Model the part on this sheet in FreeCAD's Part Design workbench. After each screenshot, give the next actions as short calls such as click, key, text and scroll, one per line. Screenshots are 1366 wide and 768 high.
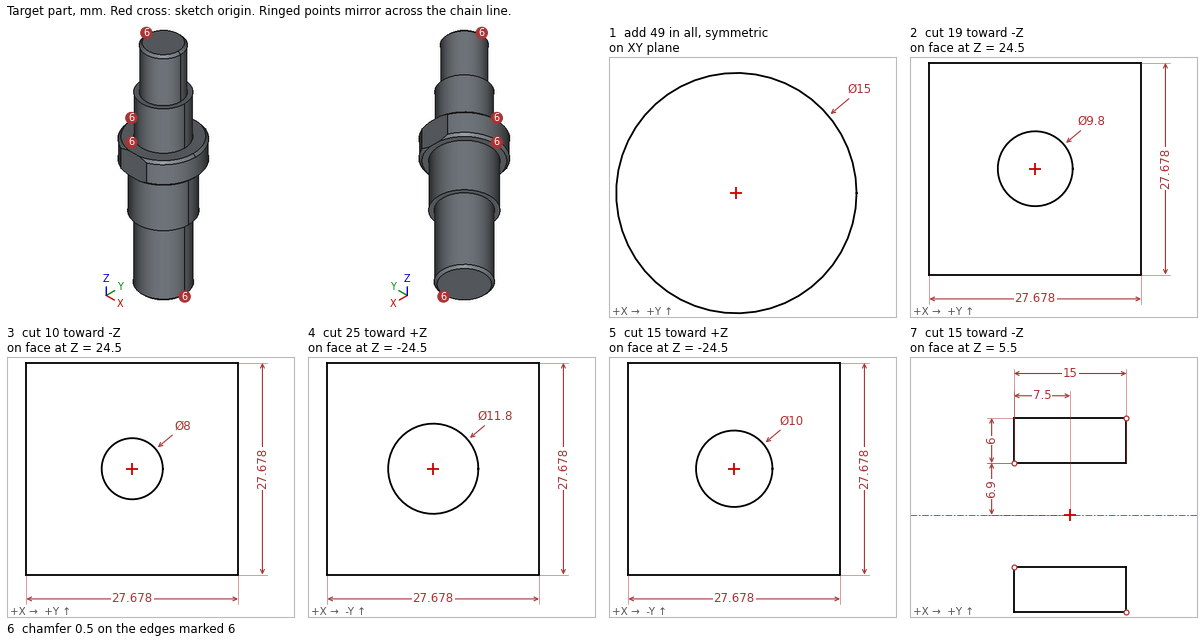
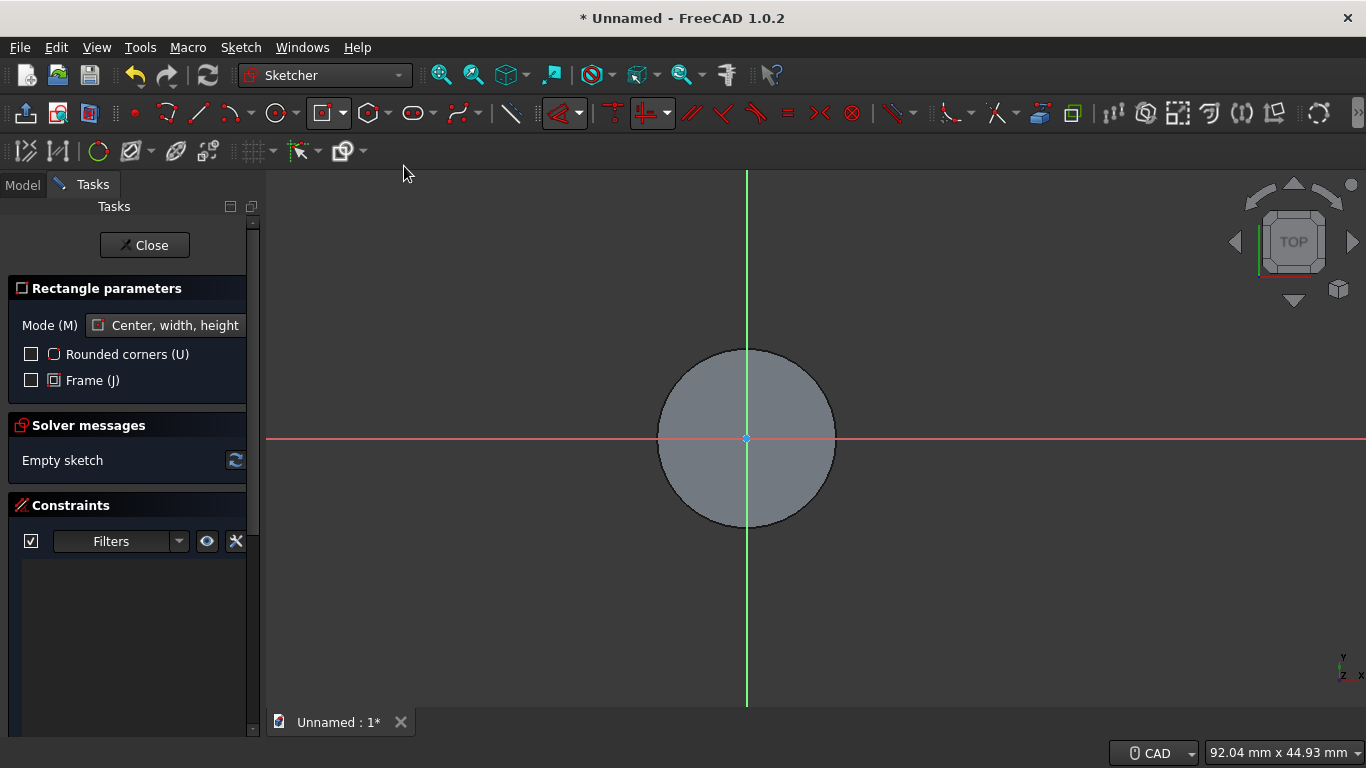
click(747, 438)
click(912, 273)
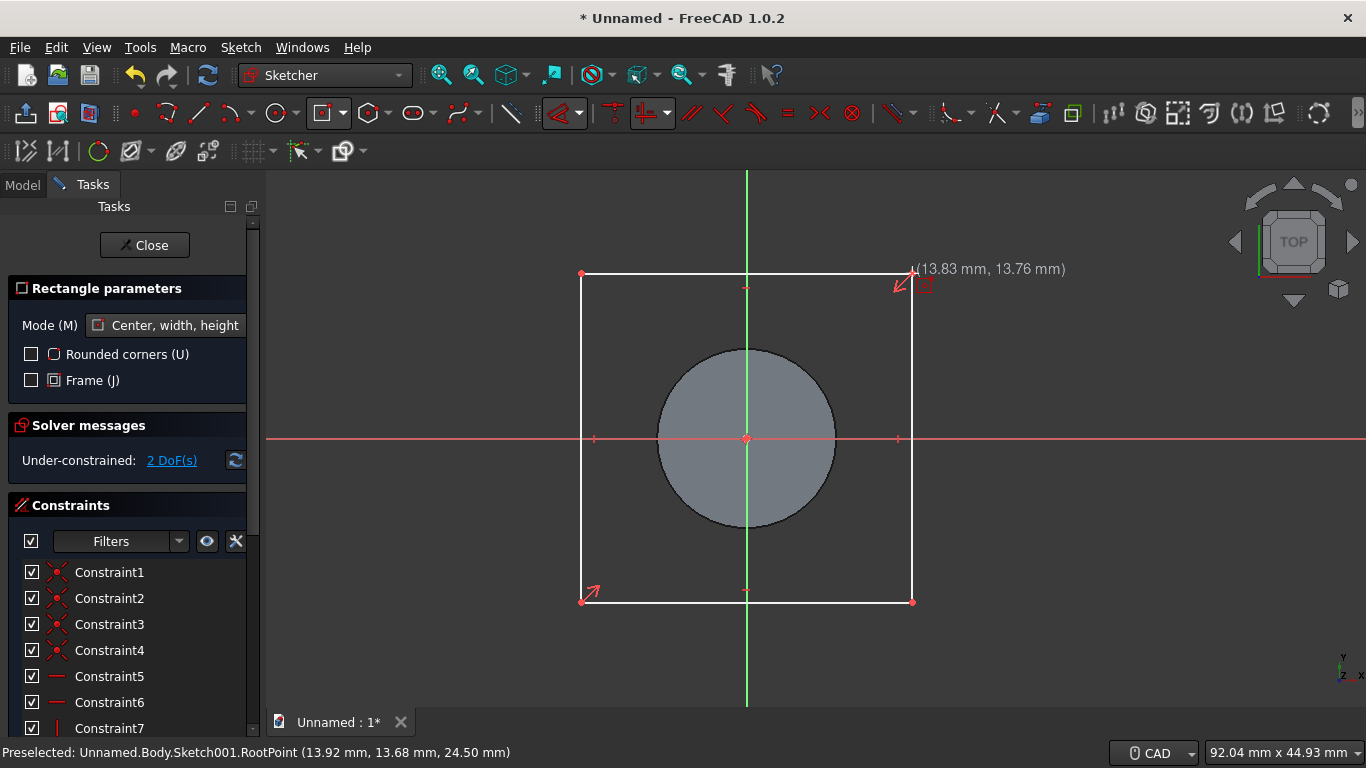
click(276, 114)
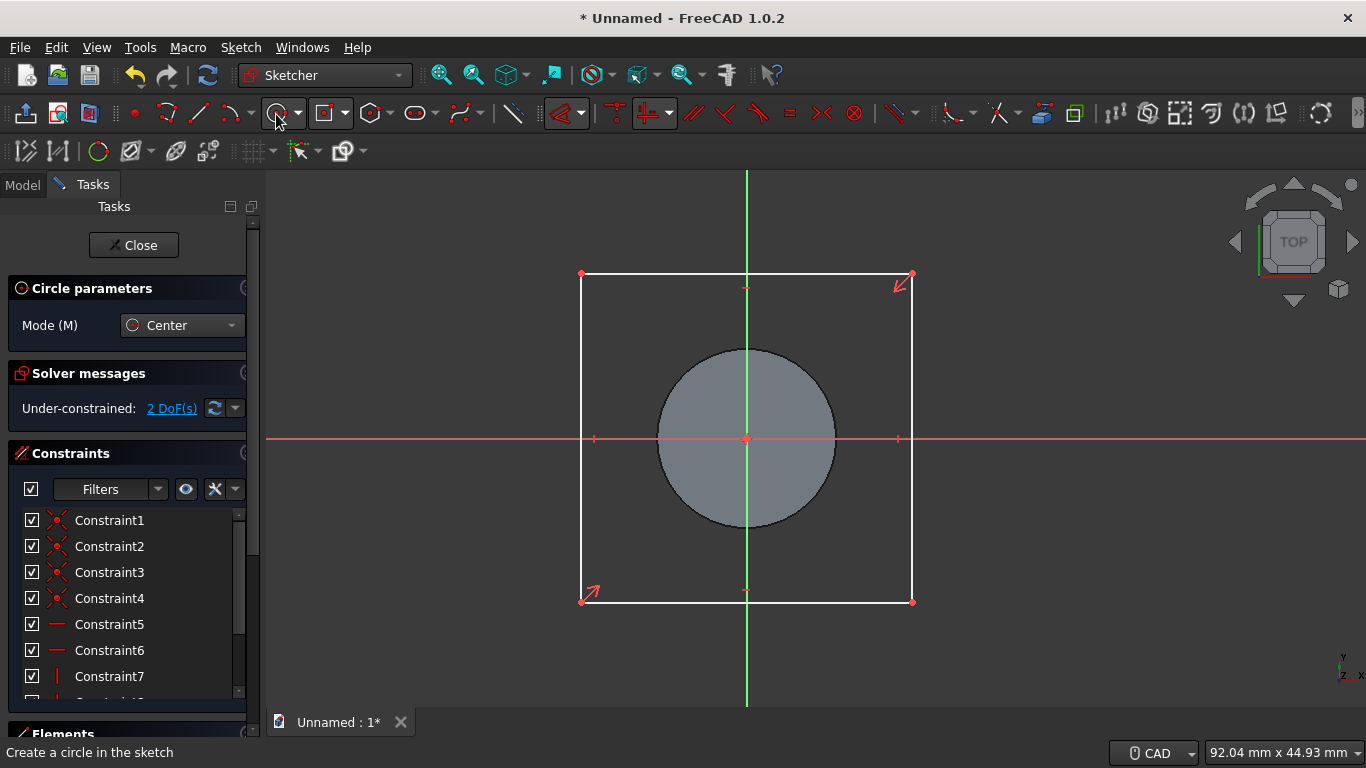
click(747, 438)
click(788, 397)
key(Escape)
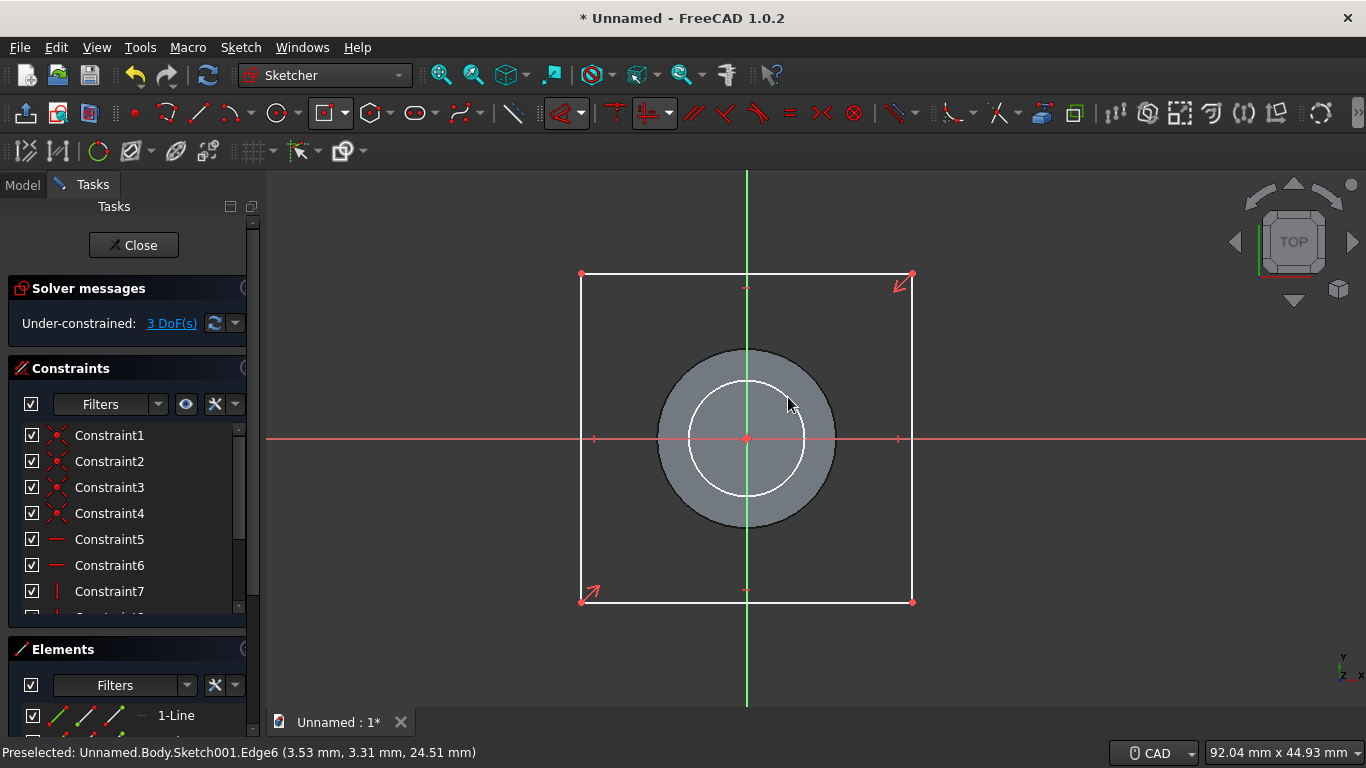
click(787, 397)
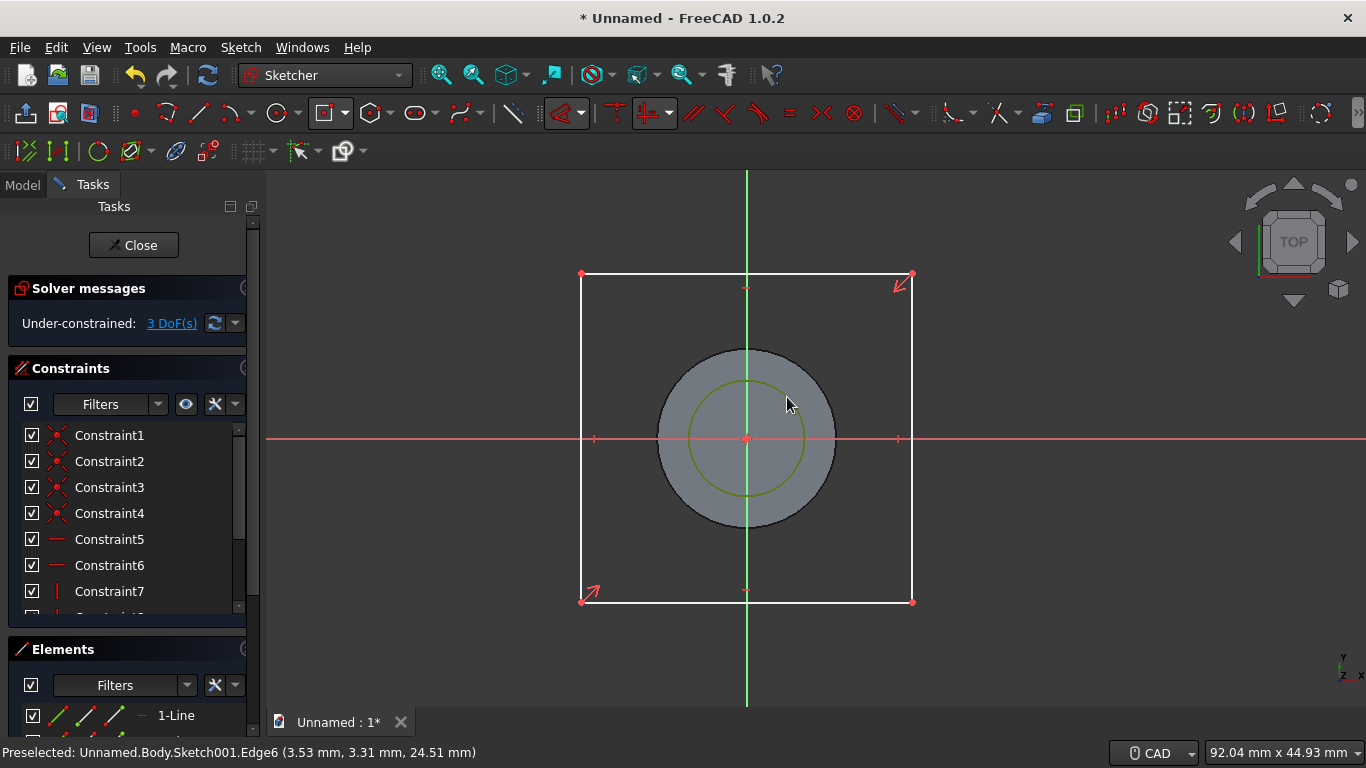
click(584, 114)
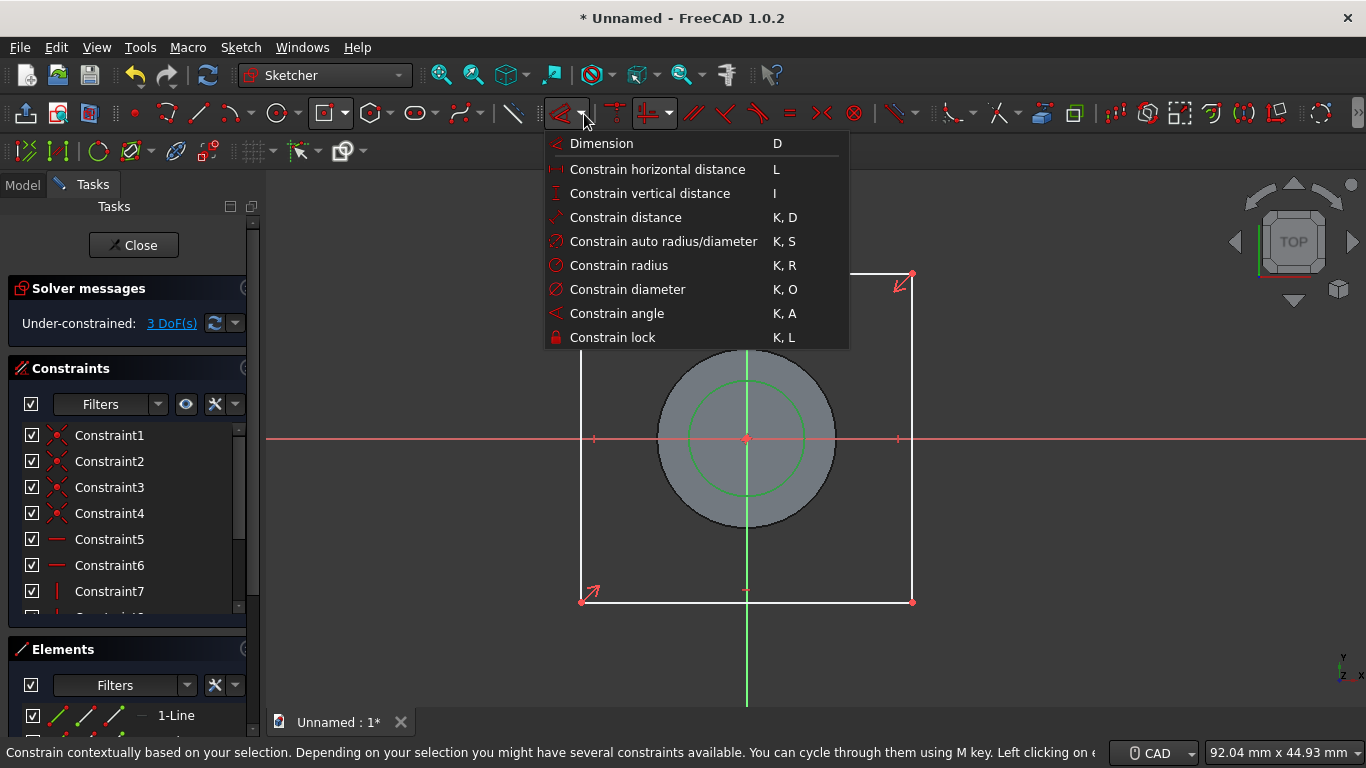
click(697, 289)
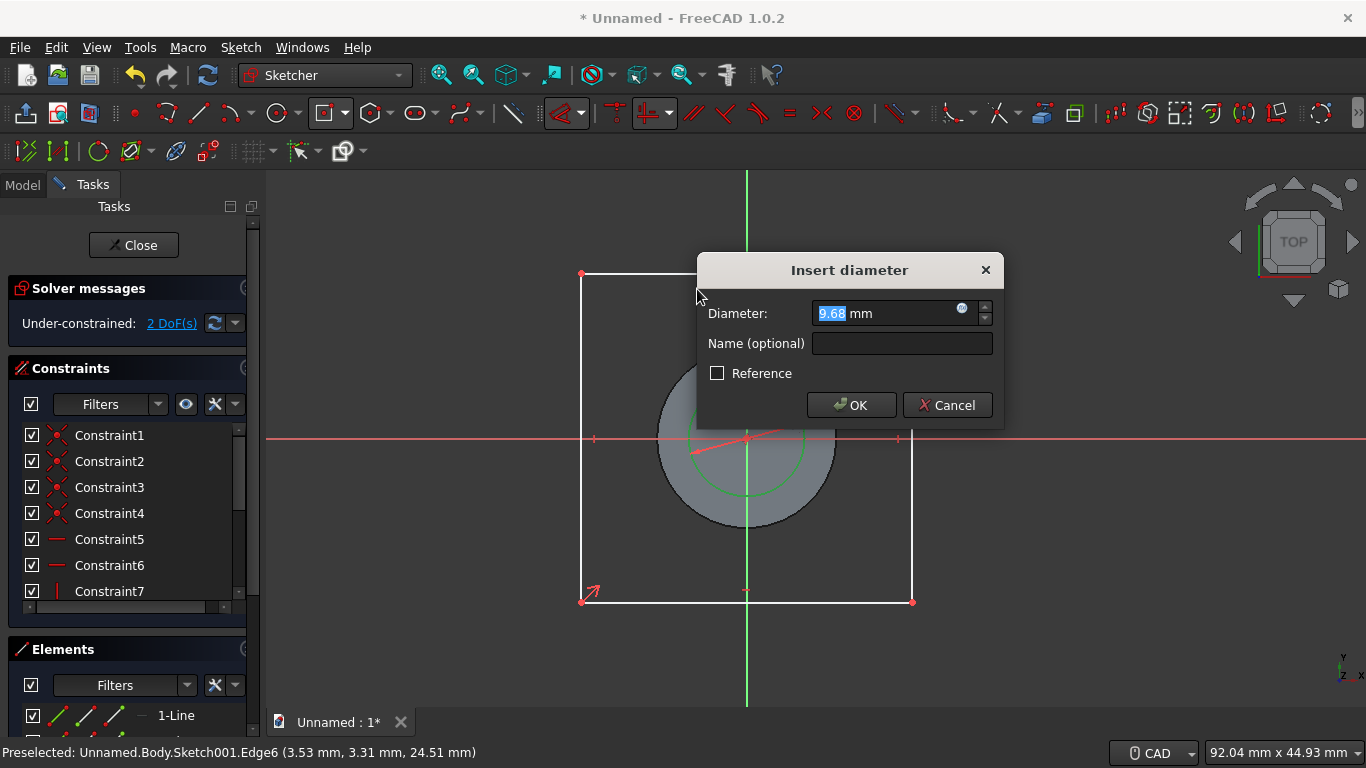
text(9.8)
key(Return)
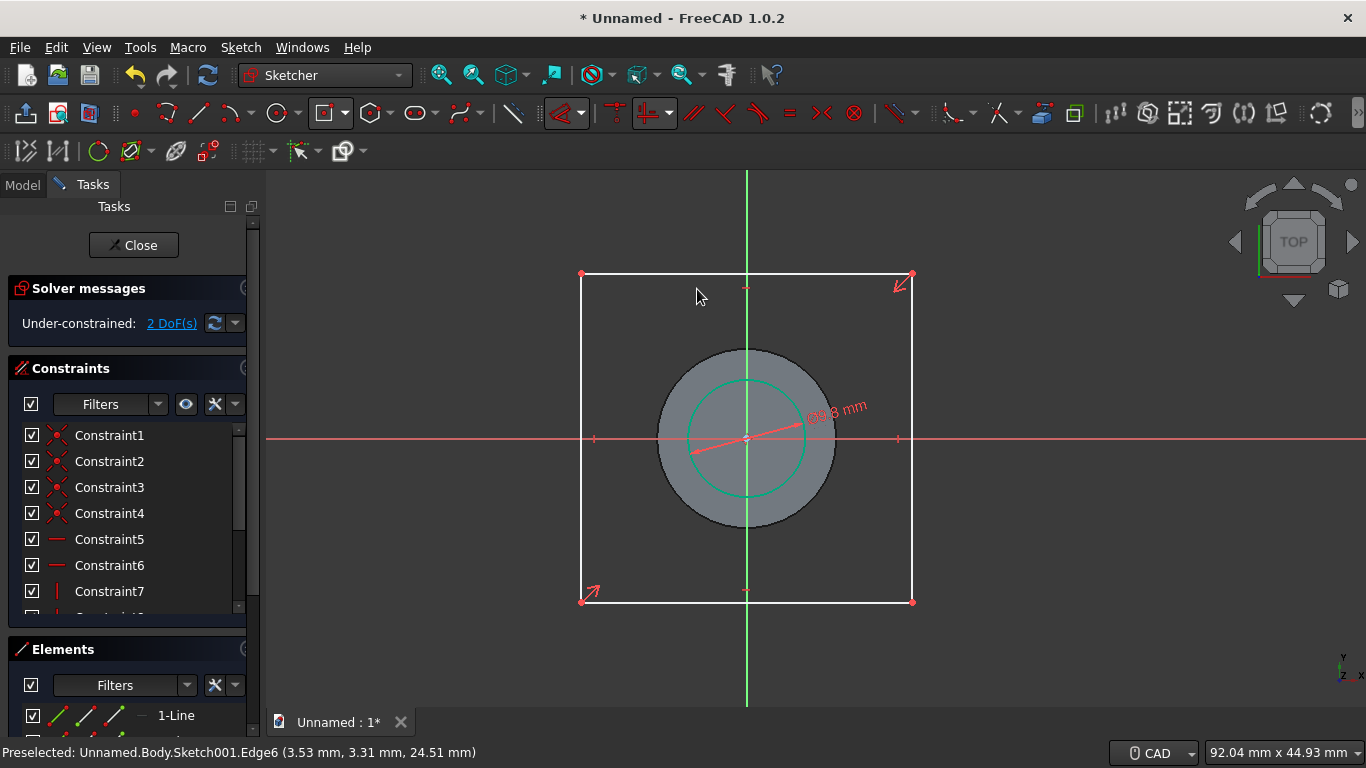
click(681, 603)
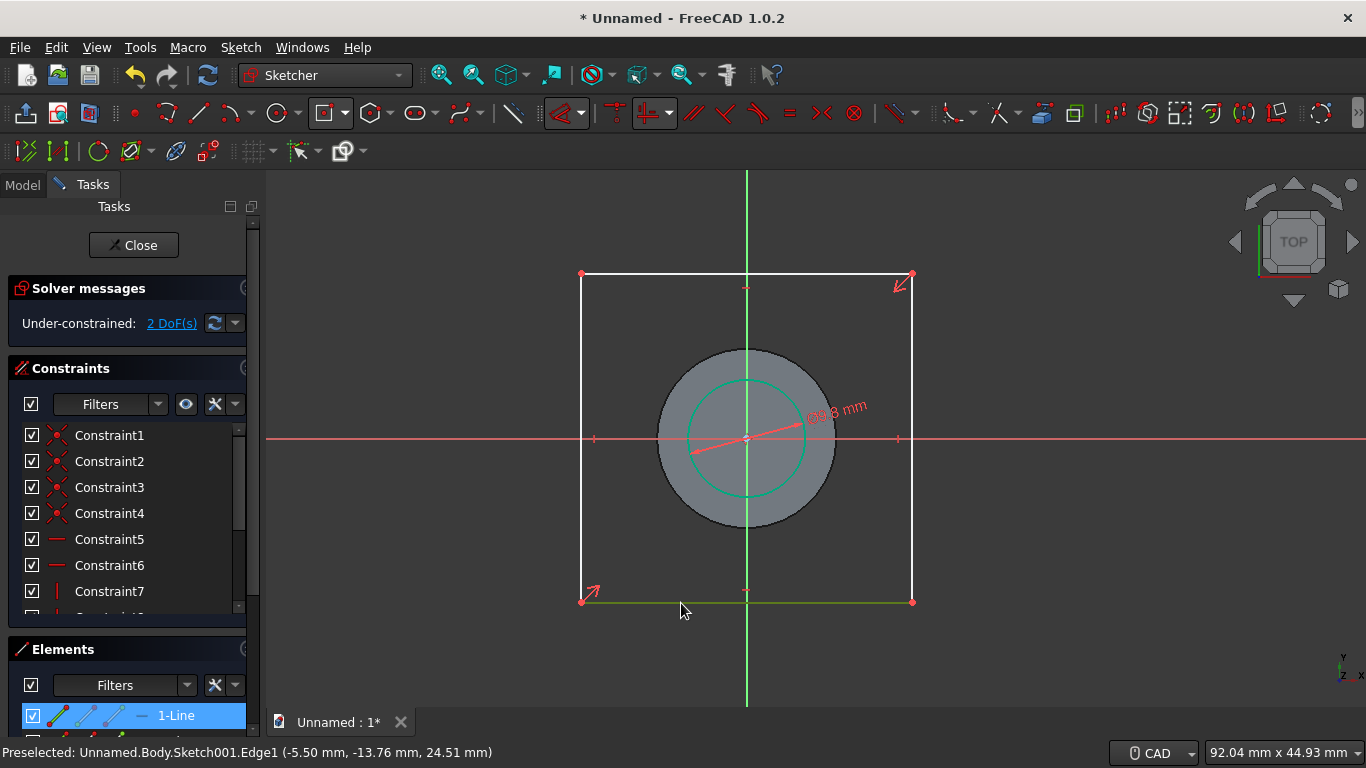
key(l)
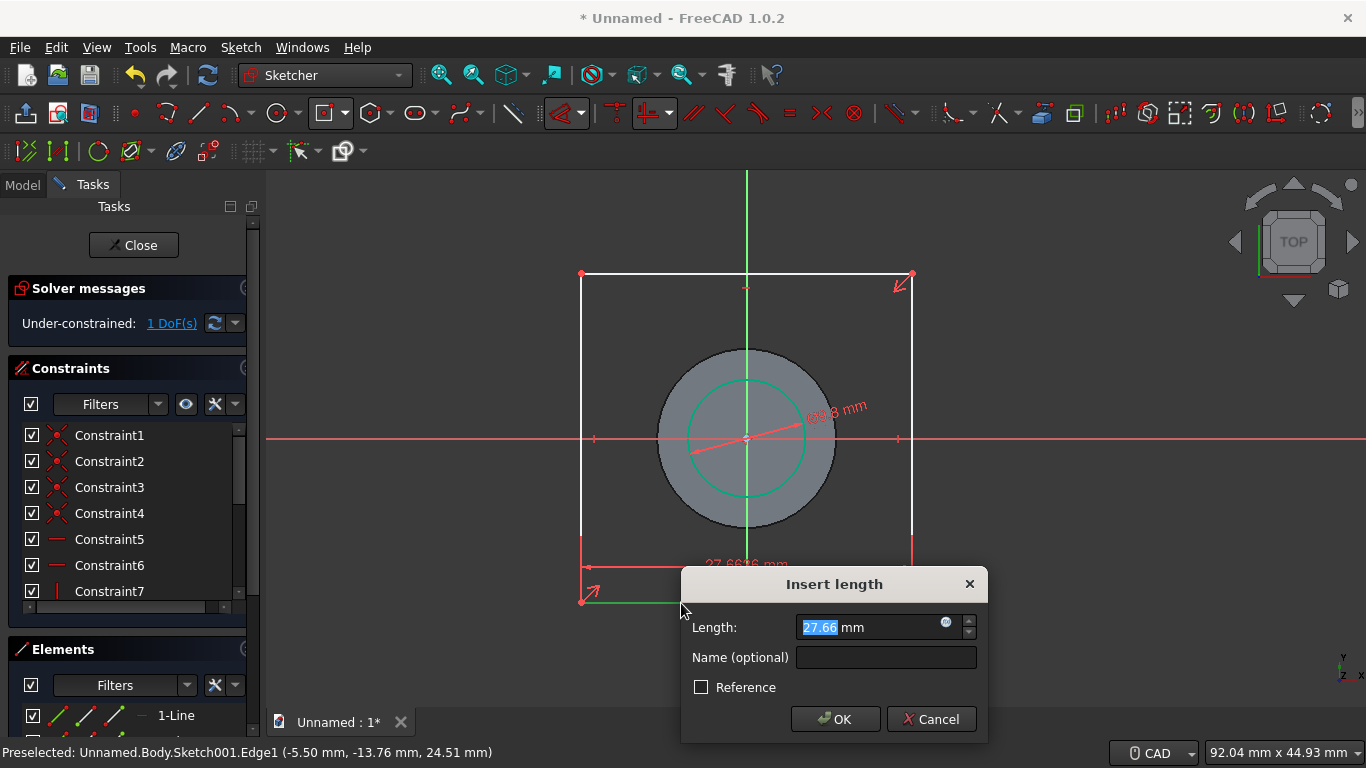
text(27.678)
key(Return)